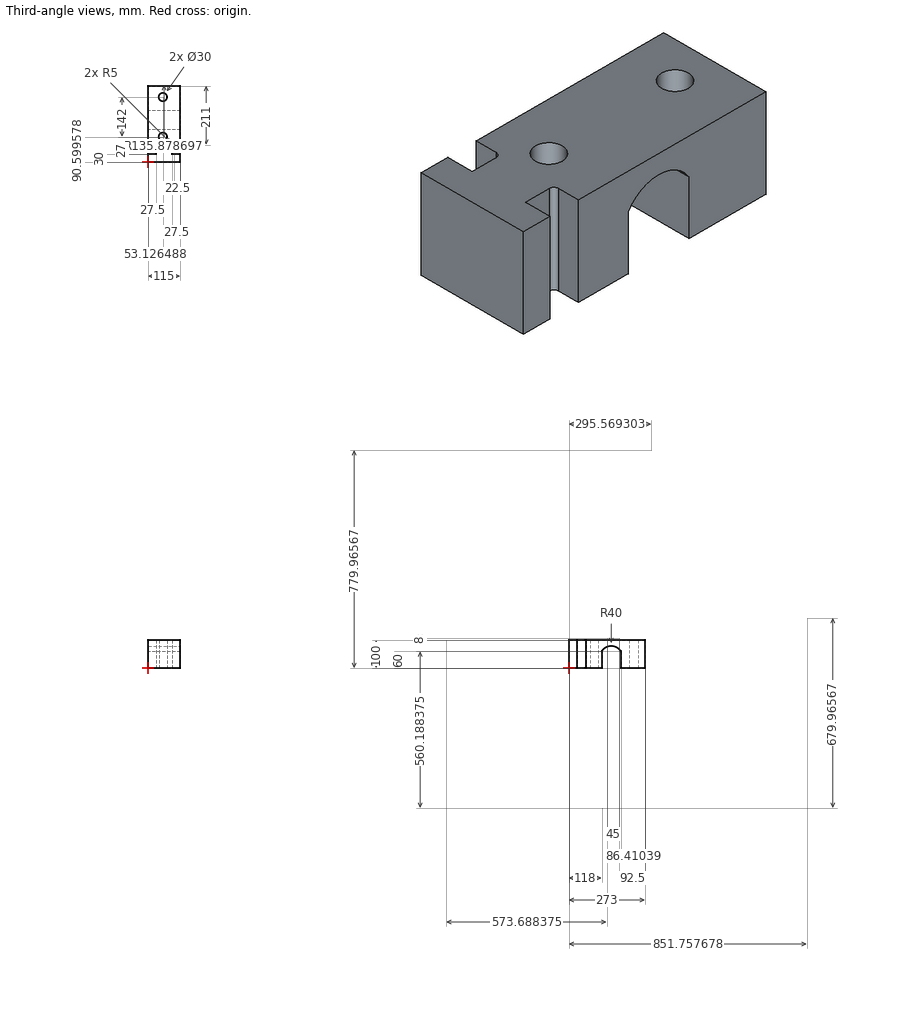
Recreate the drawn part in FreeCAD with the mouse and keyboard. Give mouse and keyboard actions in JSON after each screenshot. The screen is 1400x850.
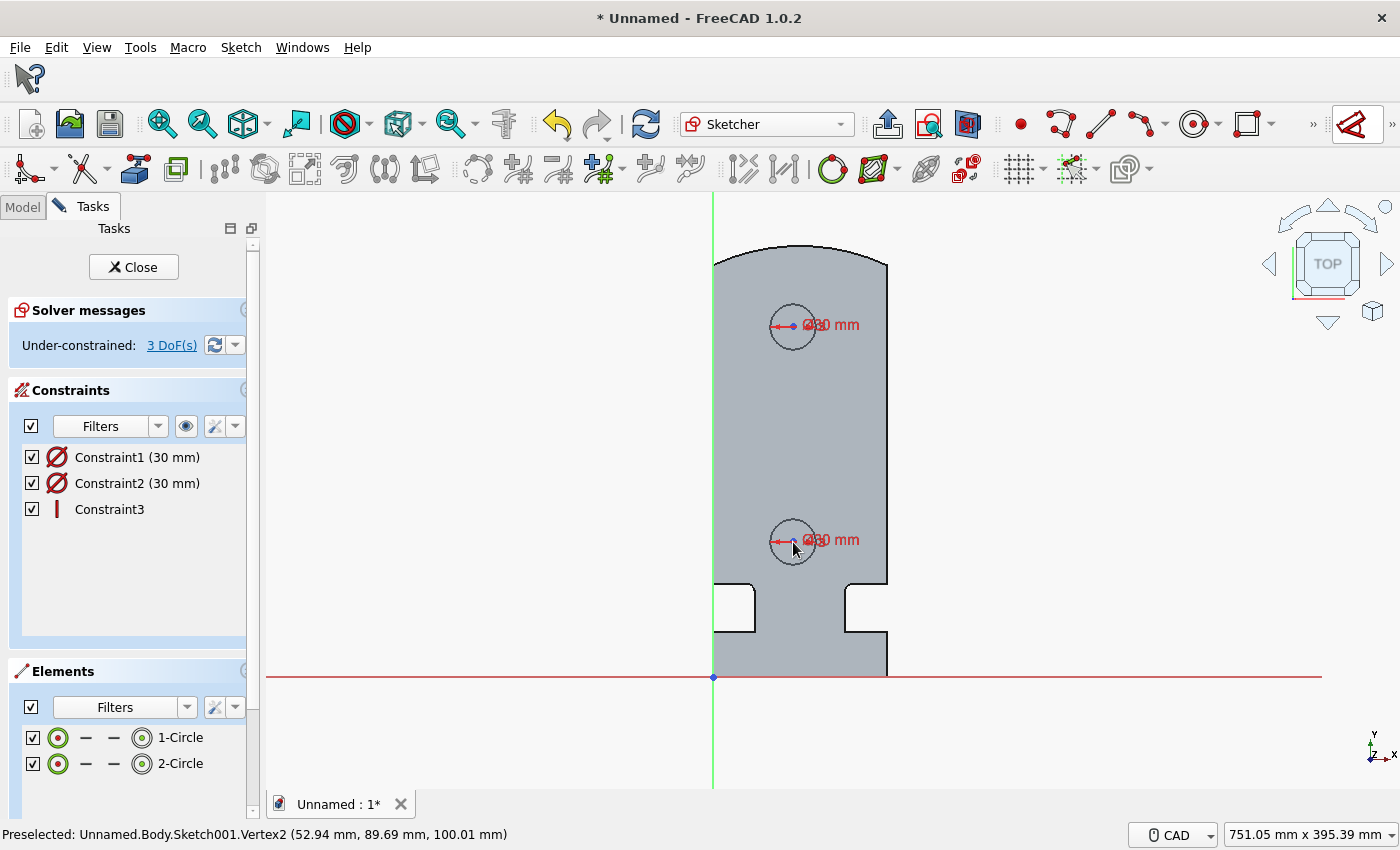
{"action": "key", "text": "d"}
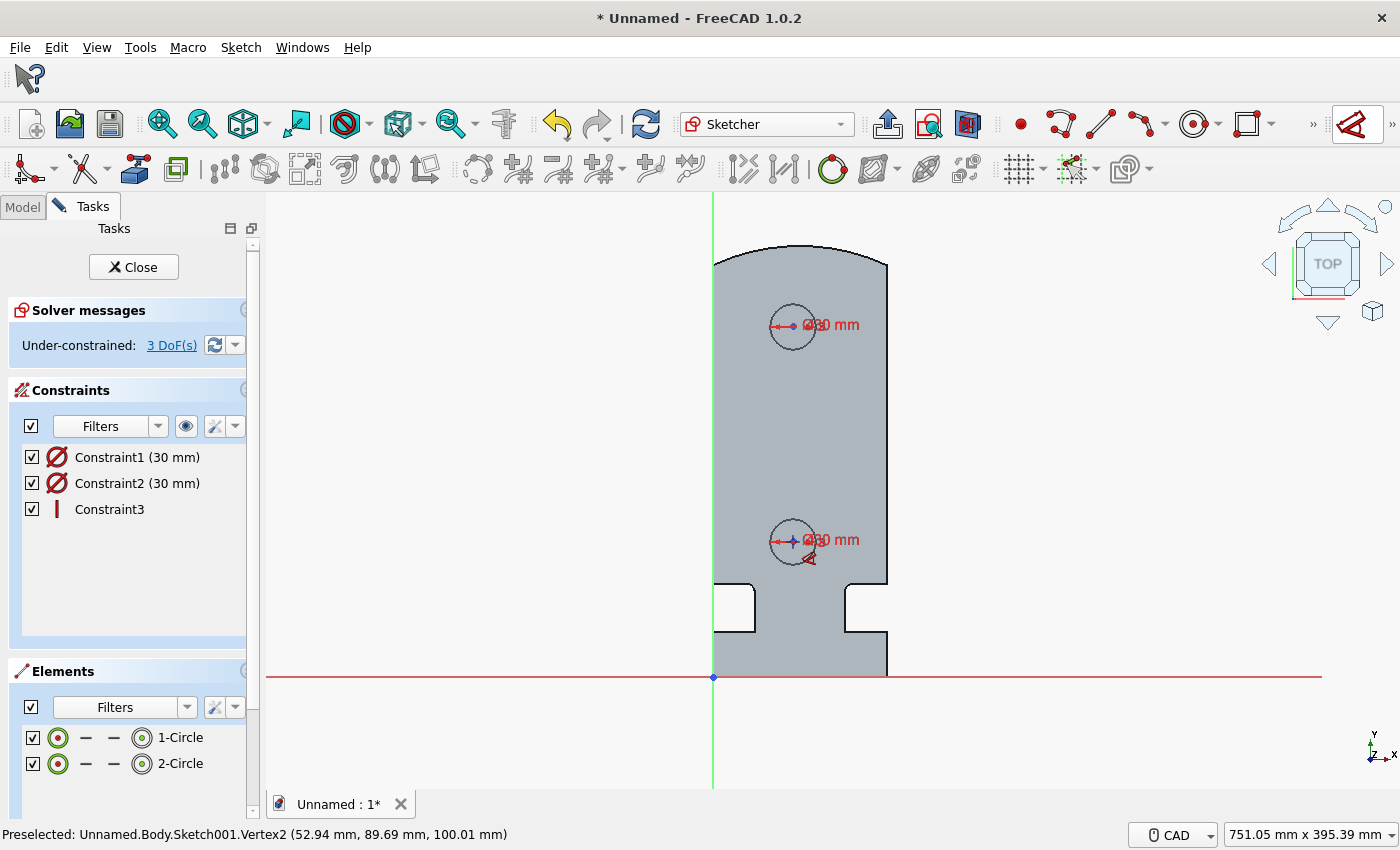
{"action": "left_click", "coordinate": [793, 327]}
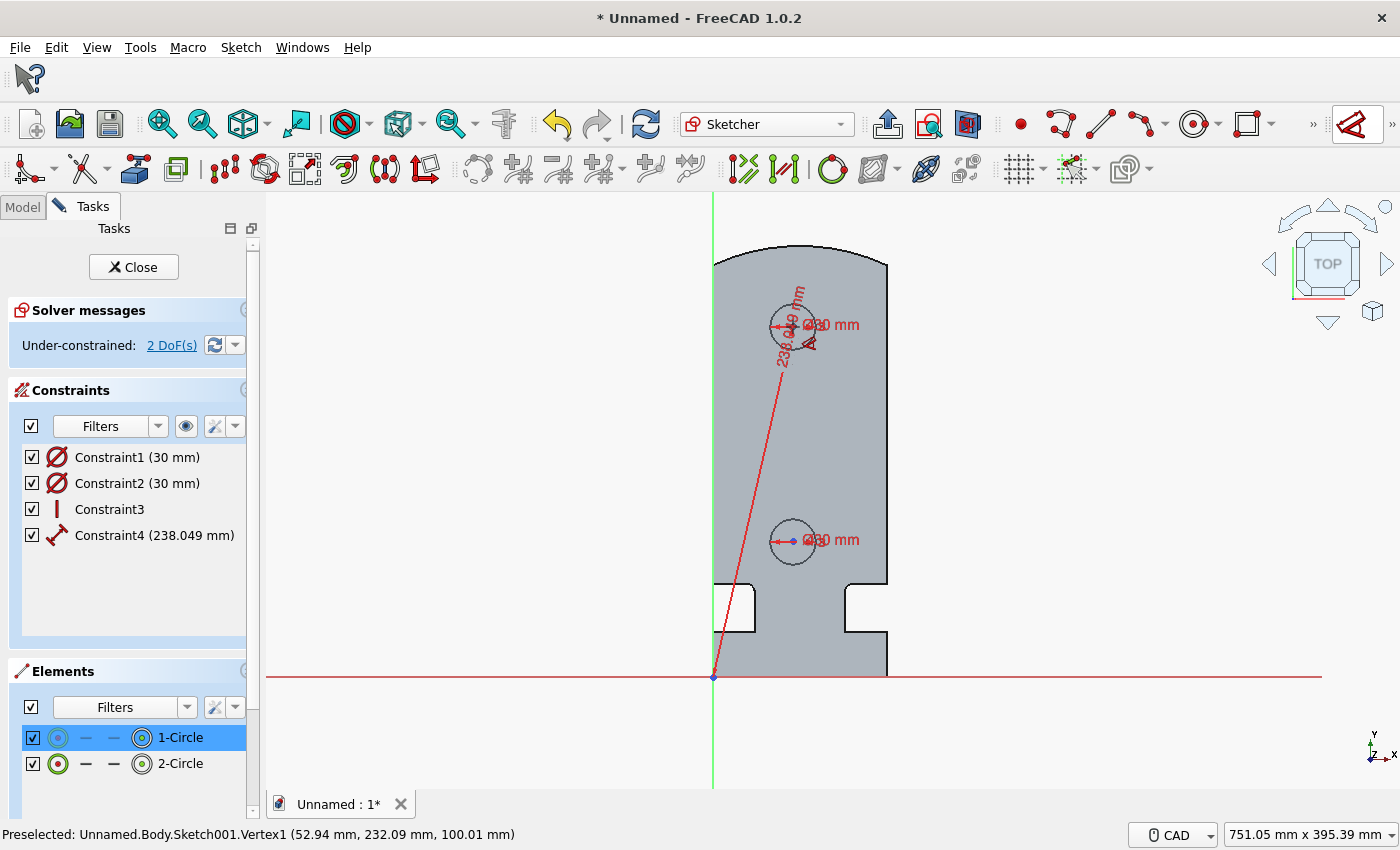
{"action": "left_click", "coordinate": [793, 542]}
{"action": "left_click", "coordinate": [827, 435]}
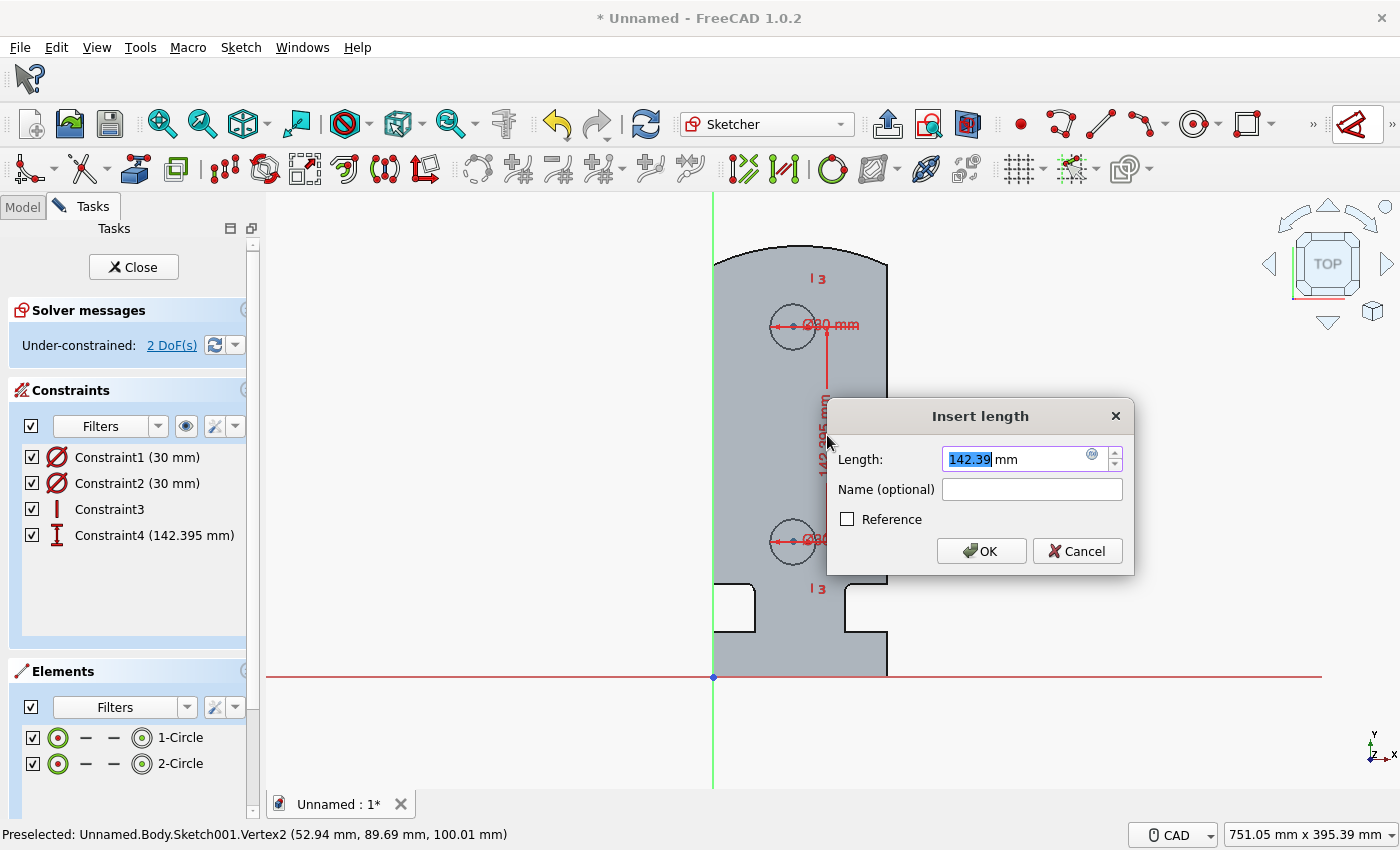
{"action": "type", "text": "142"}
{"action": "key", "text": "Return"}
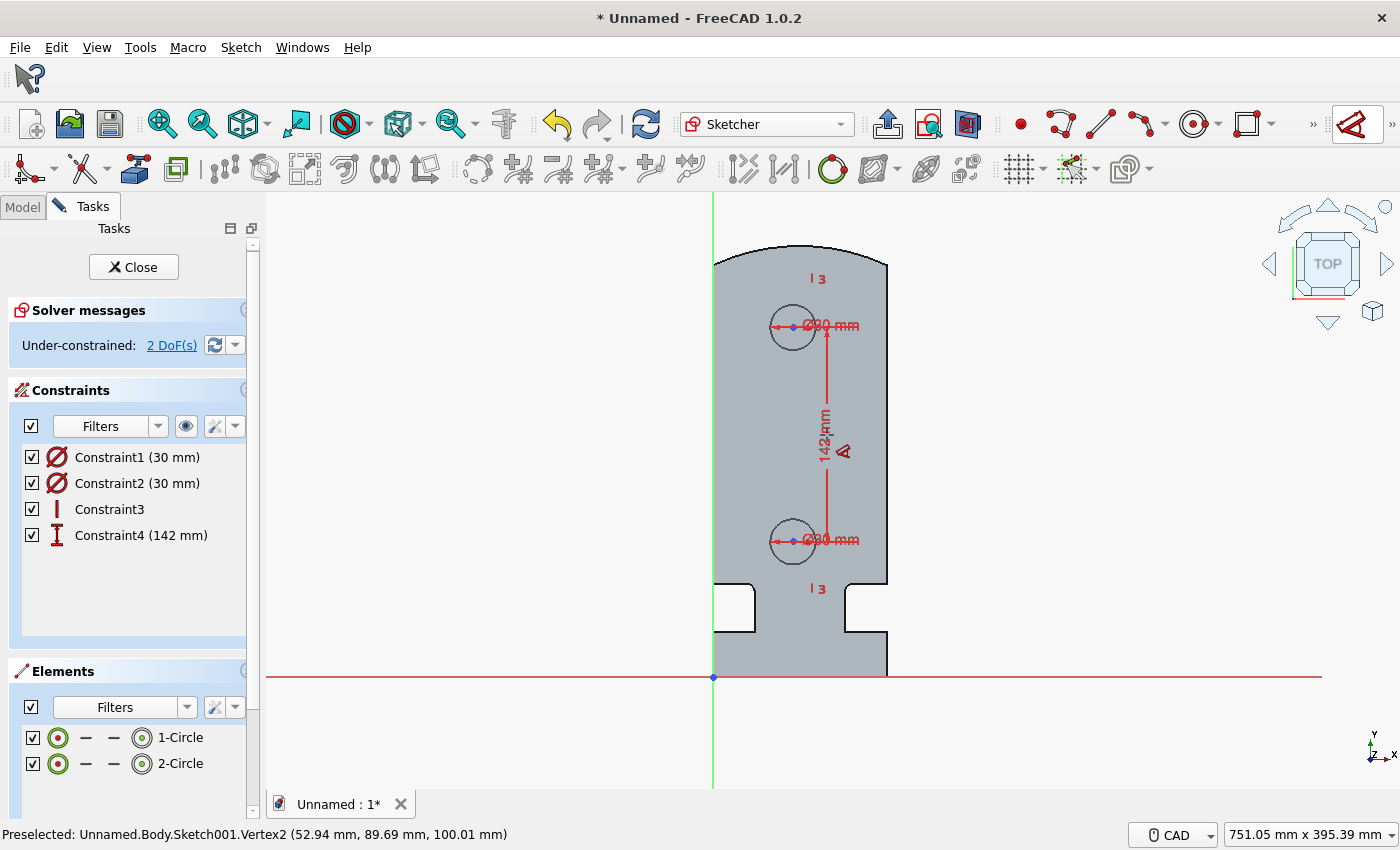
{"action": "left_click", "coordinate": [793, 327]}
{"action": "left_click", "coordinate": [753, 711]}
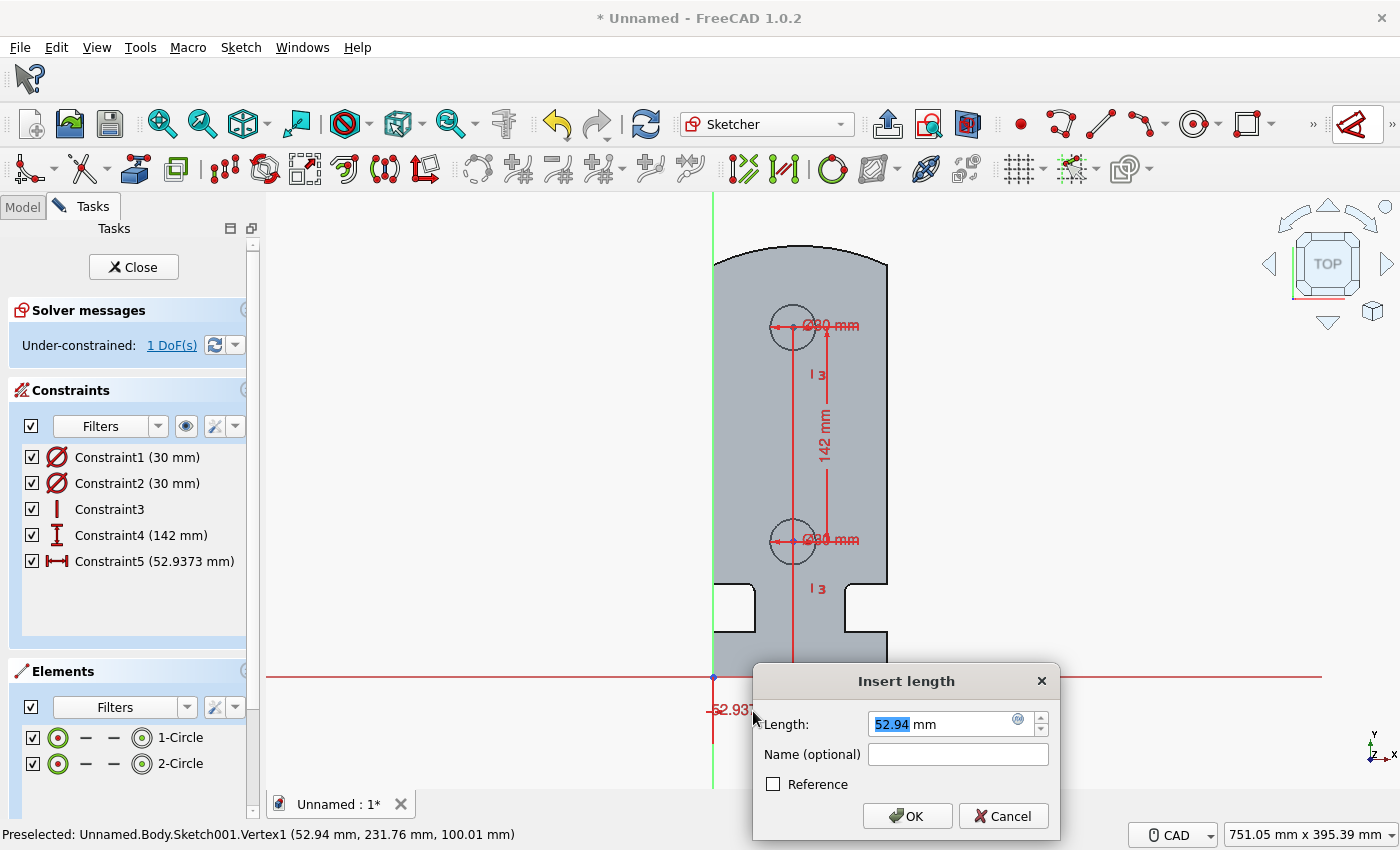
{"action": "type", "text": "53.126488"}
{"action": "key", "text": "Return"}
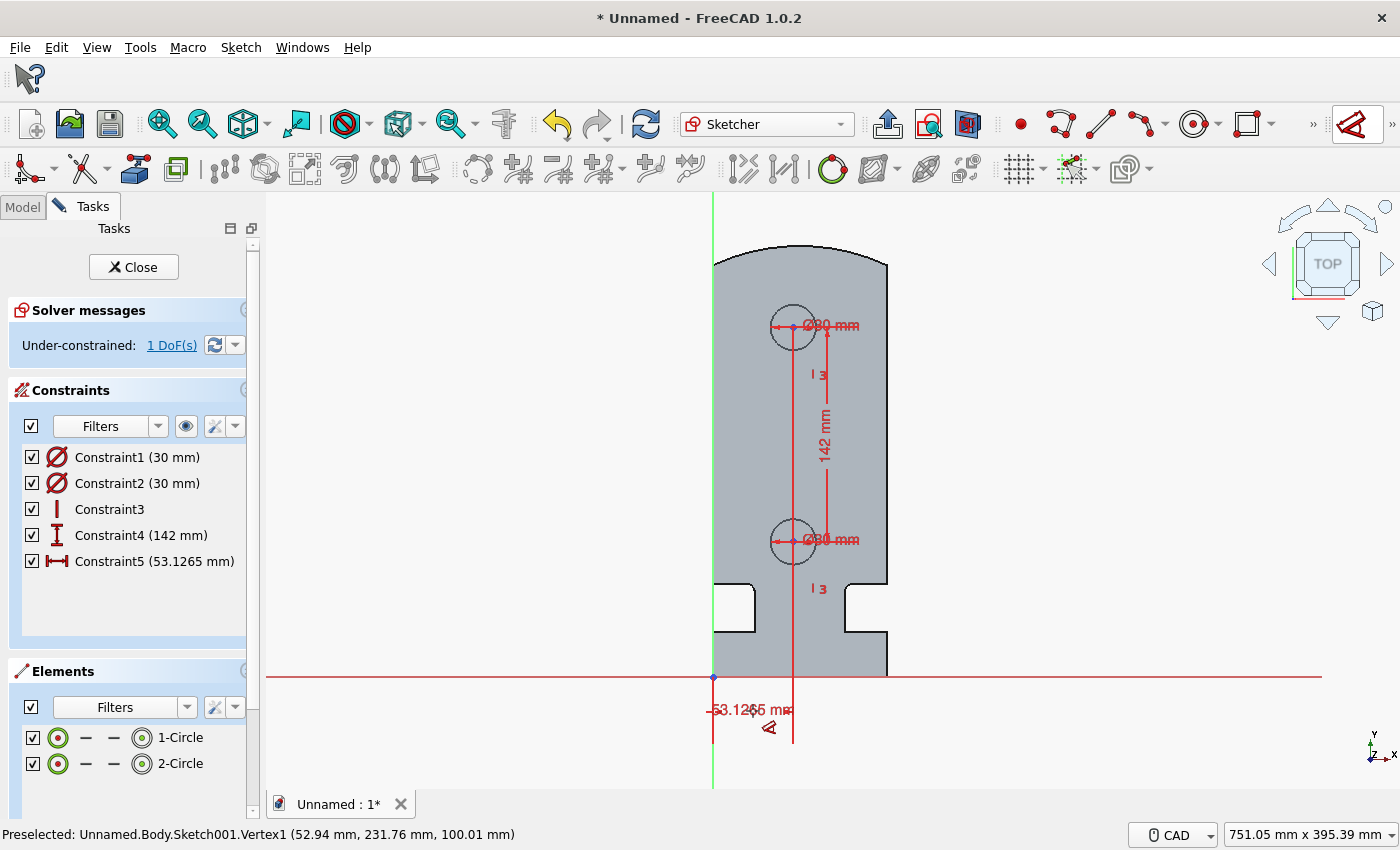
{"action": "left_click", "coordinate": [793, 542]}
{"action": "left_click", "coordinate": [679, 610]}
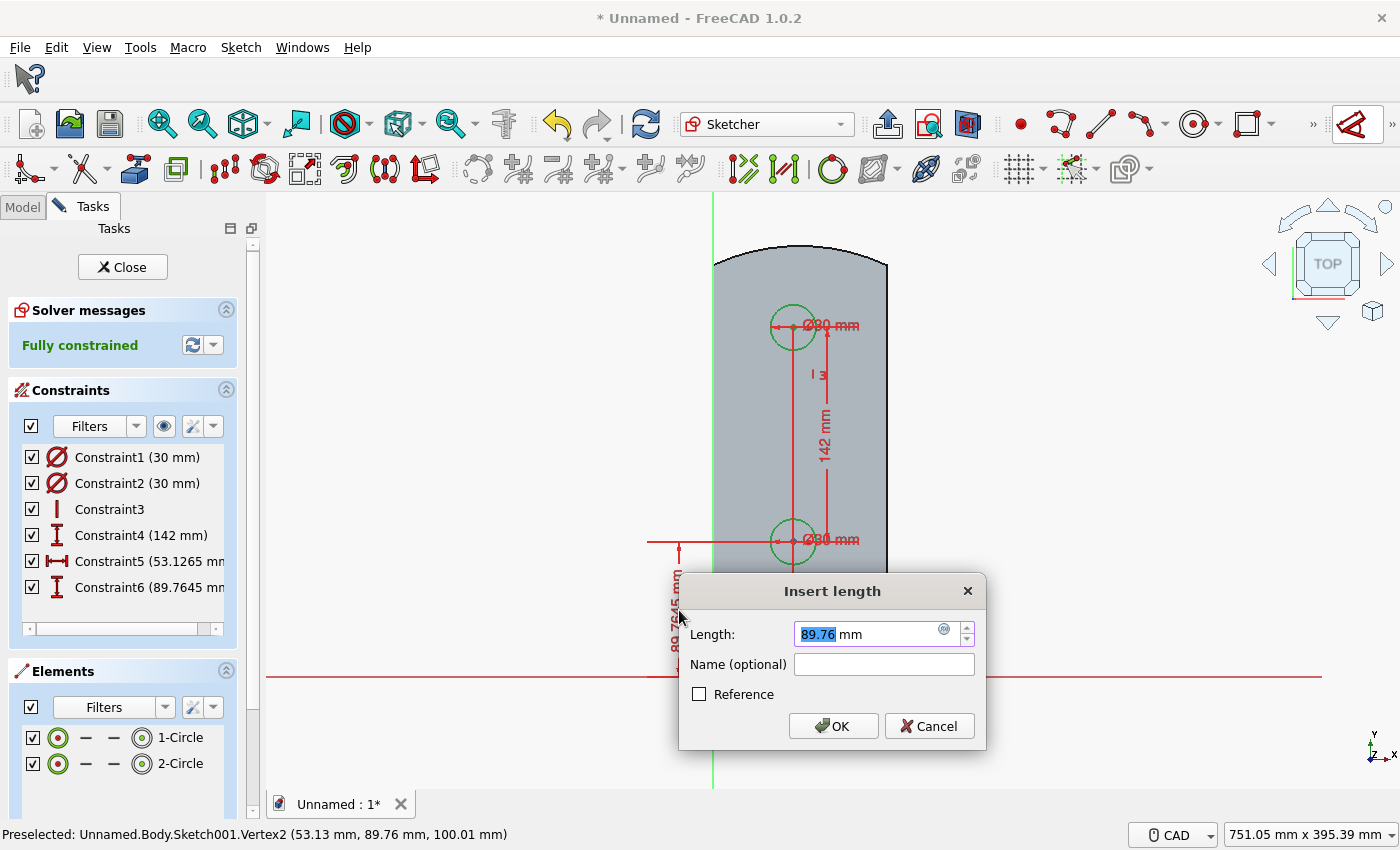
{"action": "type", "text": "90.599578"}
{"action": "key", "text": "Return"}
{"action": "key", "text": "Escape"}